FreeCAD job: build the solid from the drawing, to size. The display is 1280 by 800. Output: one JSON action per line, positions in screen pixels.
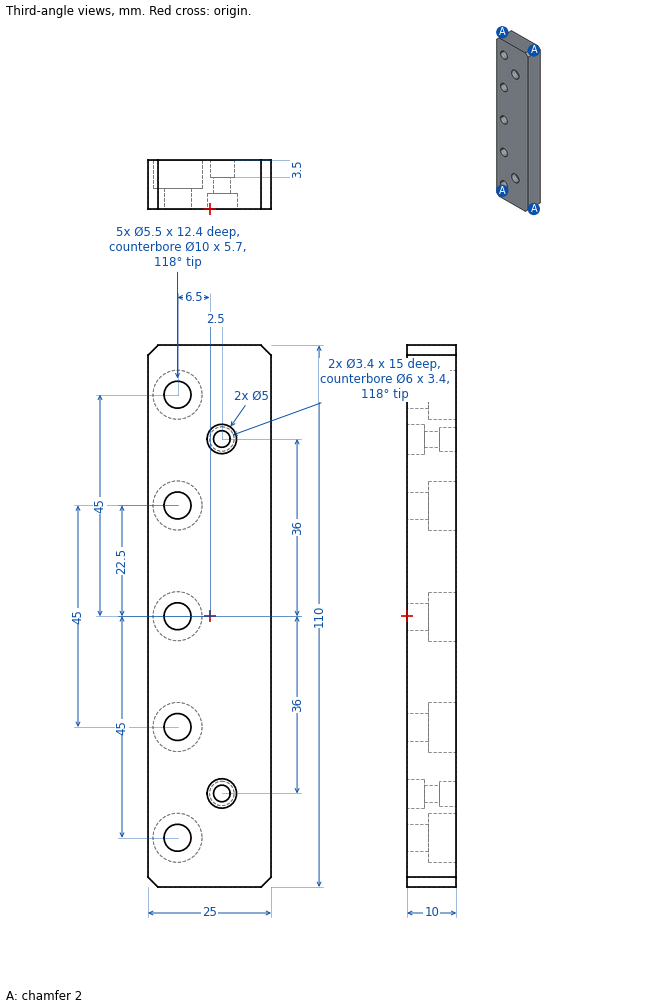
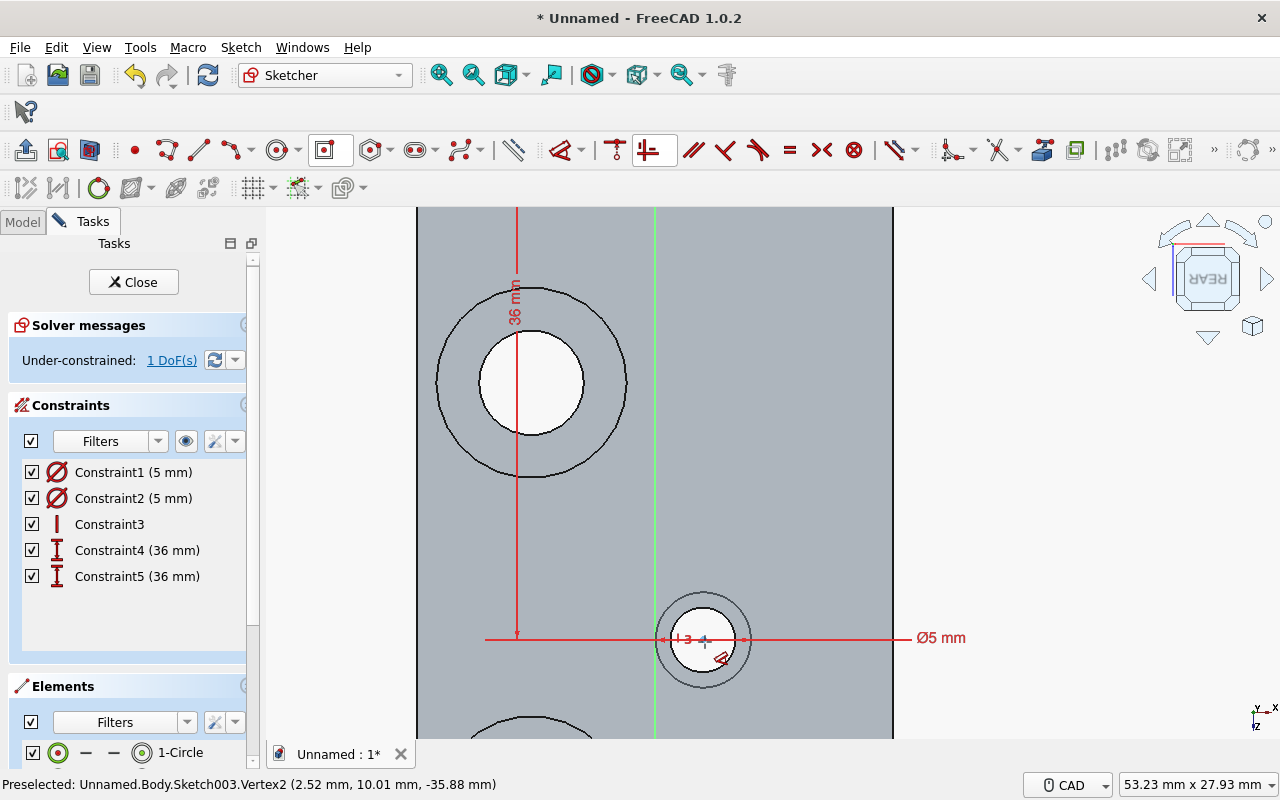
{"action": "left_click", "coordinate": [703, 640]}
{"action": "left_click", "coordinate": [679, 698]}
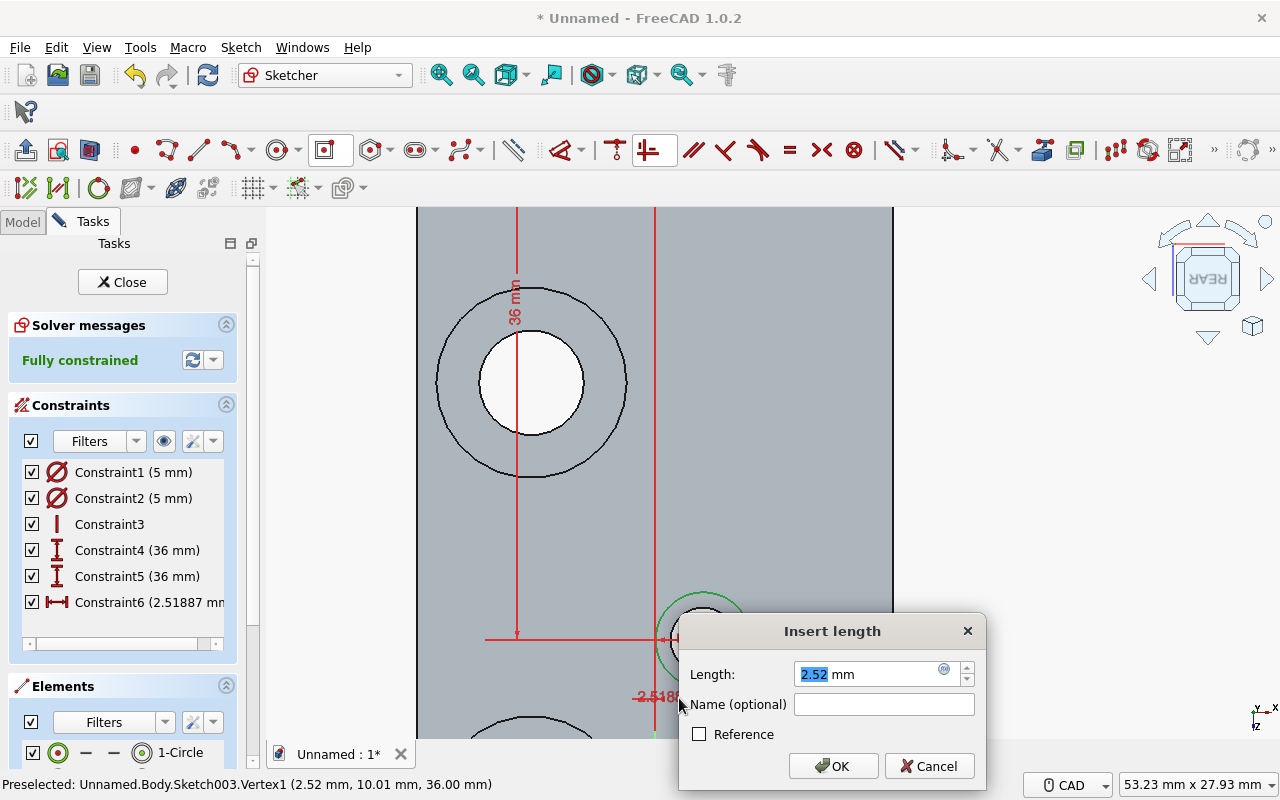
{"action": "type", "text": "2.5"}
{"action": "key", "text": "Return"}
{"action": "key", "text": "Escape"}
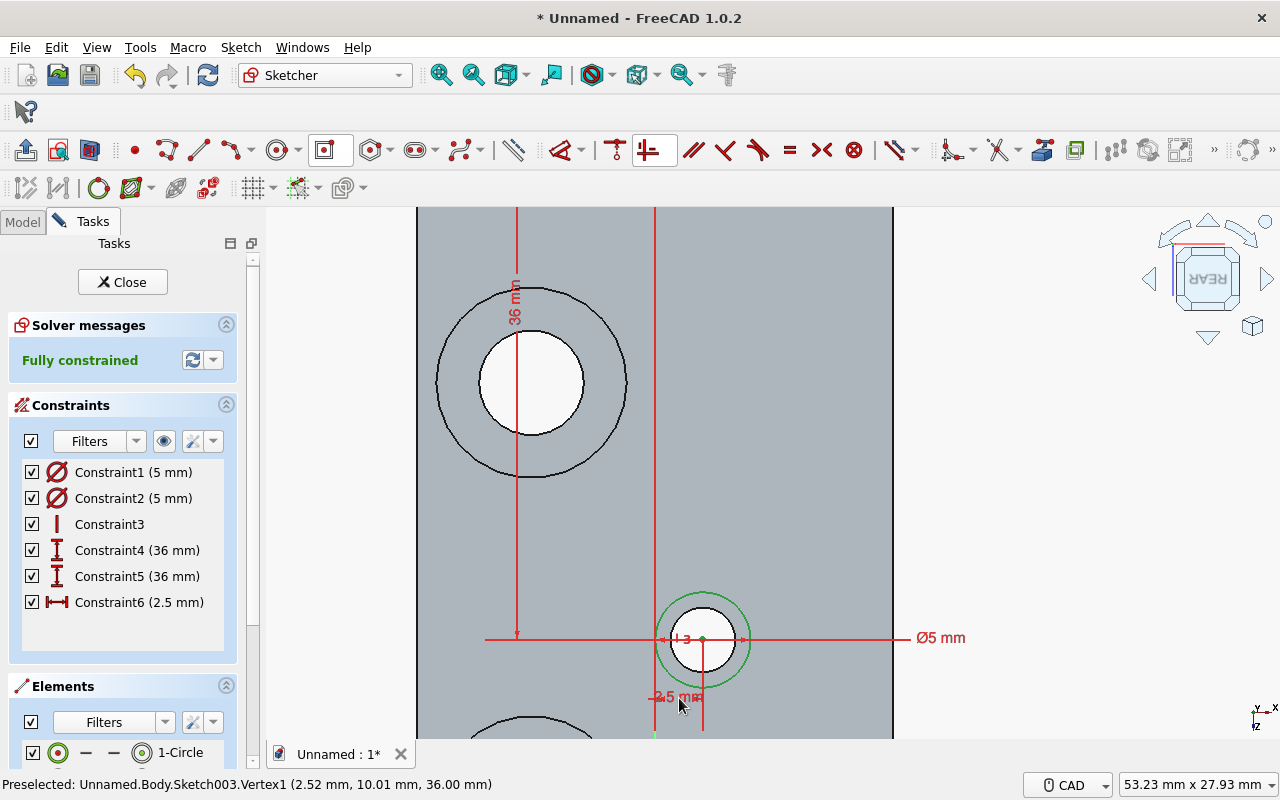
{"action": "left_click", "coordinate": [123, 282]}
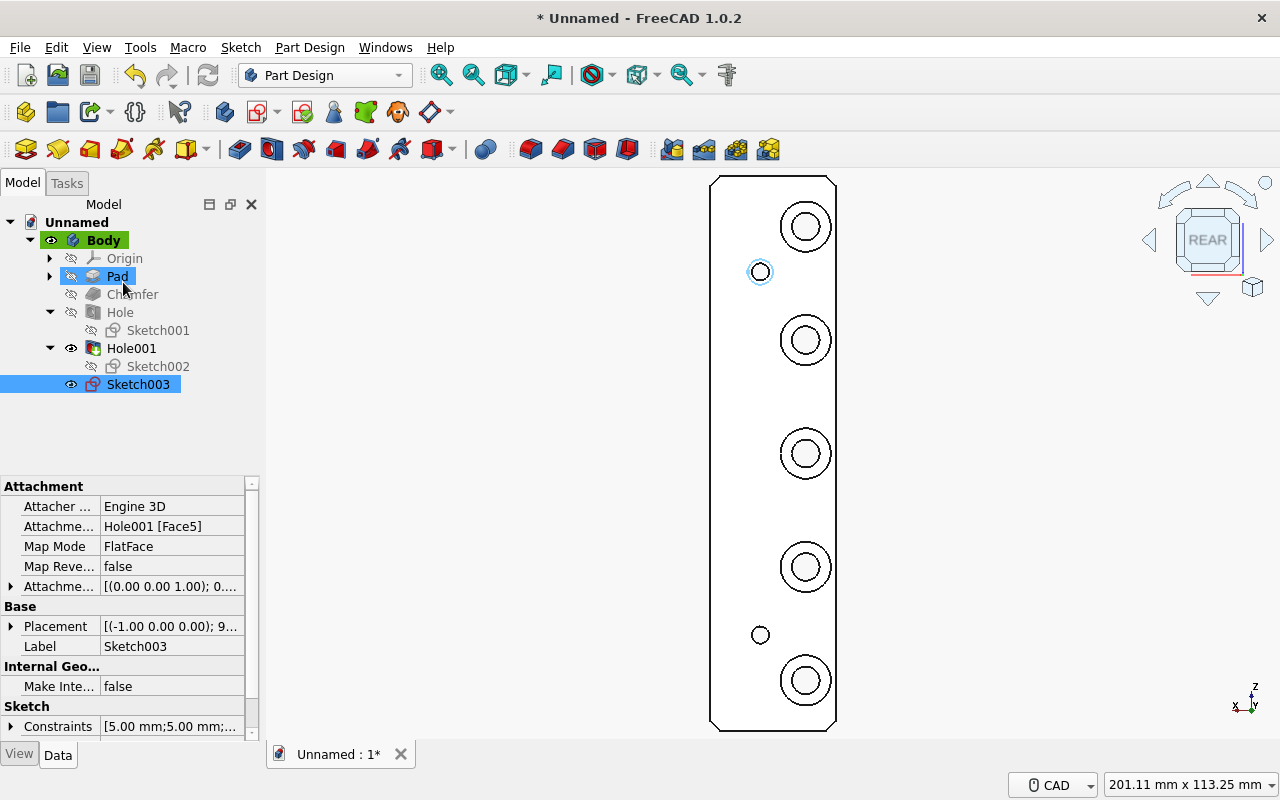
{"action": "left_click", "coordinate": [240, 150]}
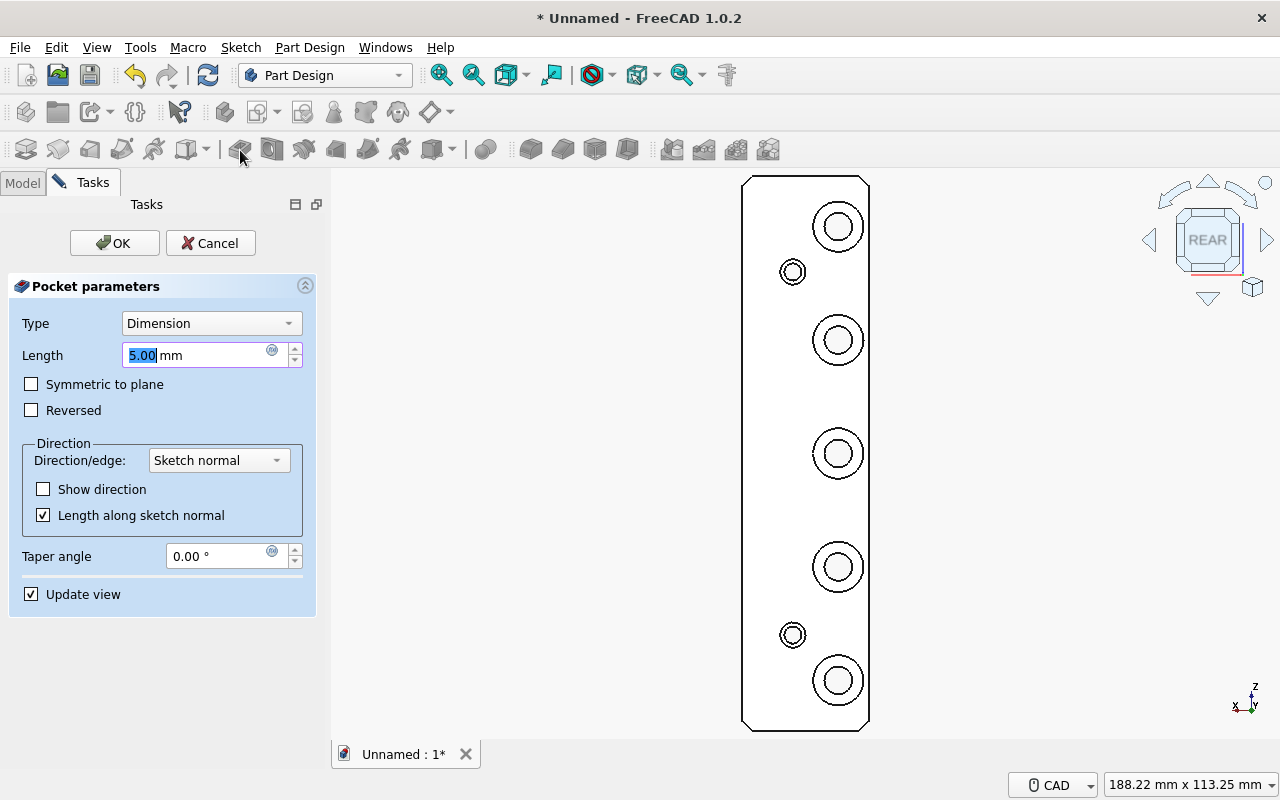
{"action": "type", "text": "3.5"}
{"action": "key", "text": "Tab"}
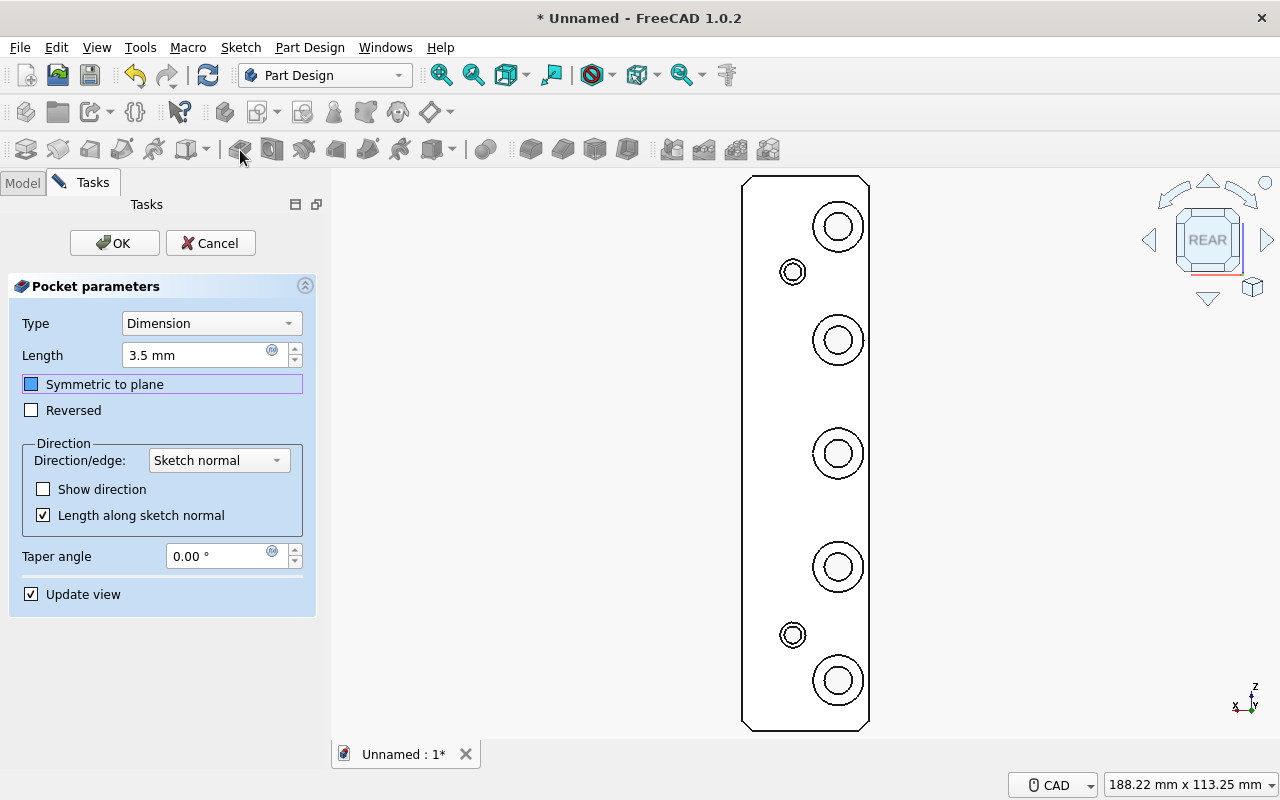
{"action": "left_click", "coordinate": [115, 243]}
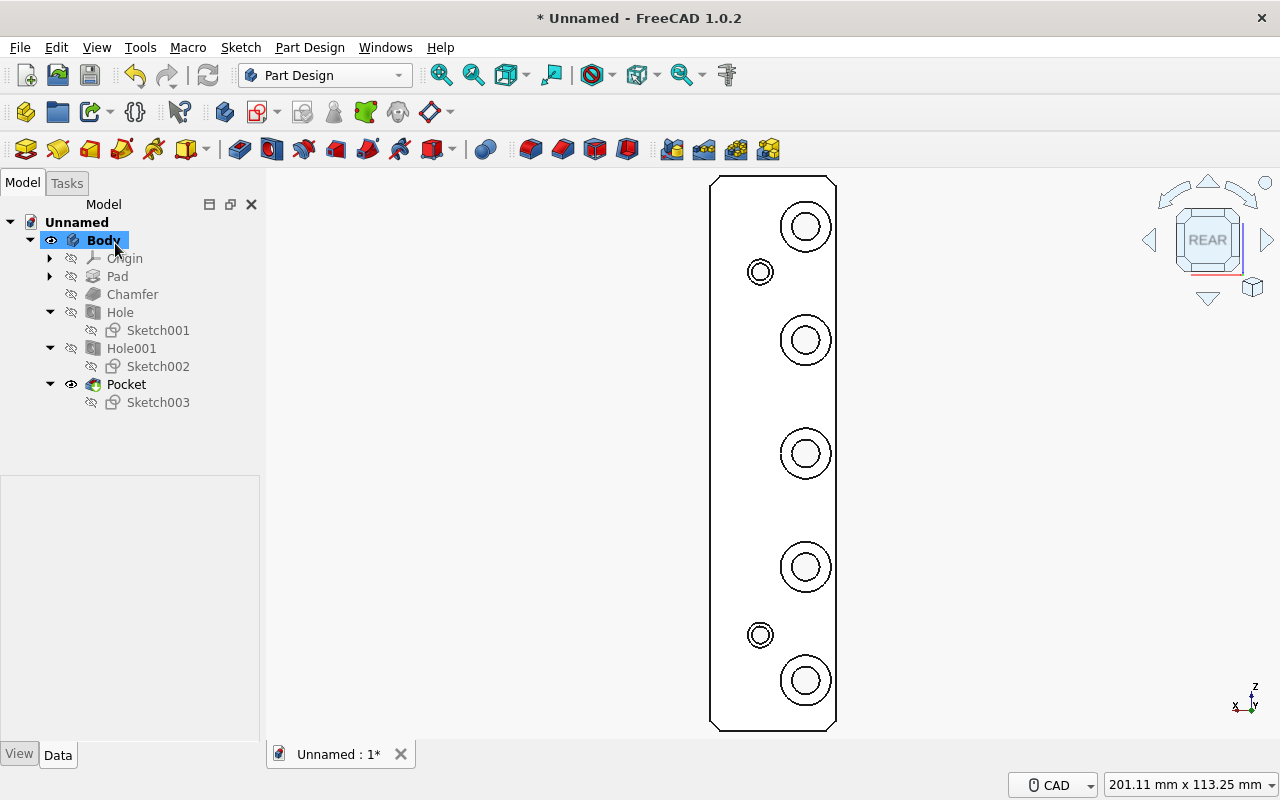
{"action": "key", "text": "0"}